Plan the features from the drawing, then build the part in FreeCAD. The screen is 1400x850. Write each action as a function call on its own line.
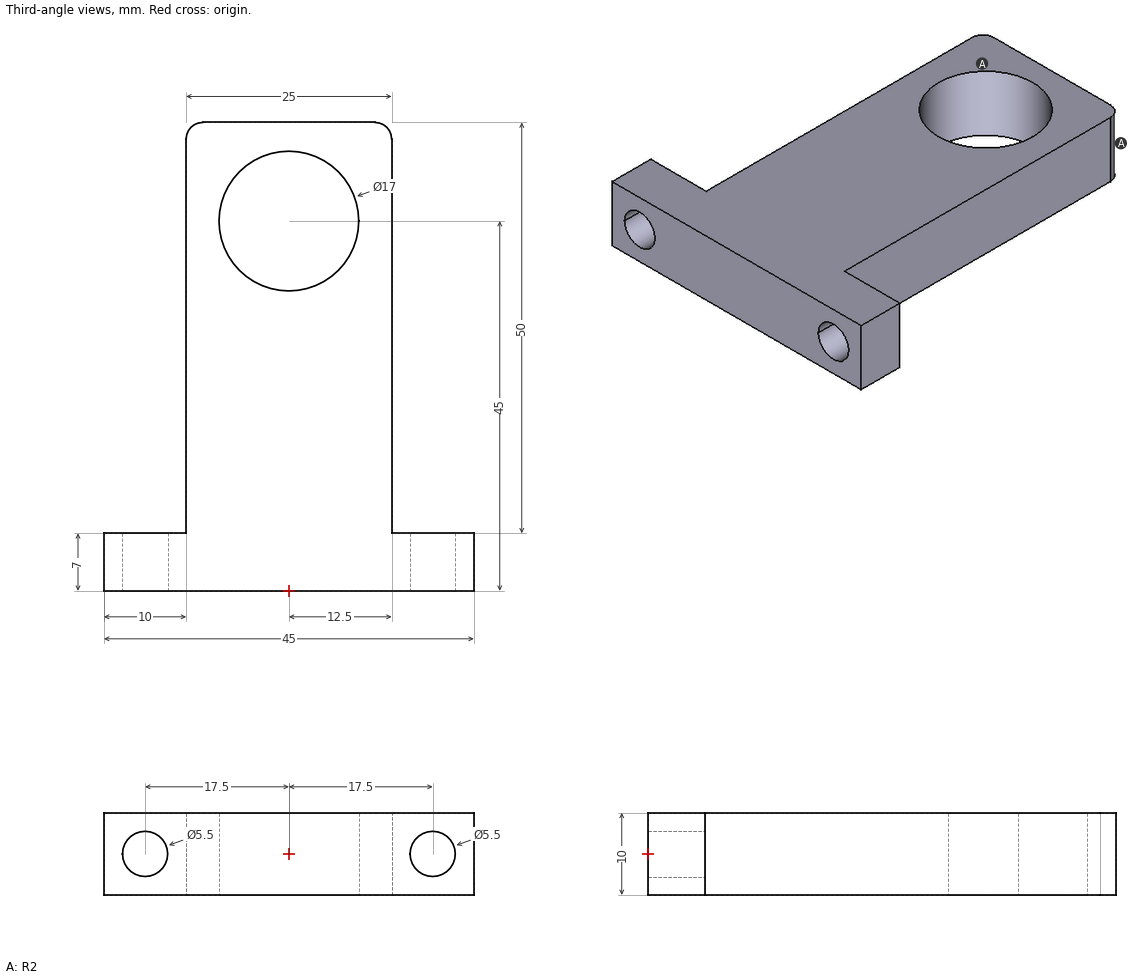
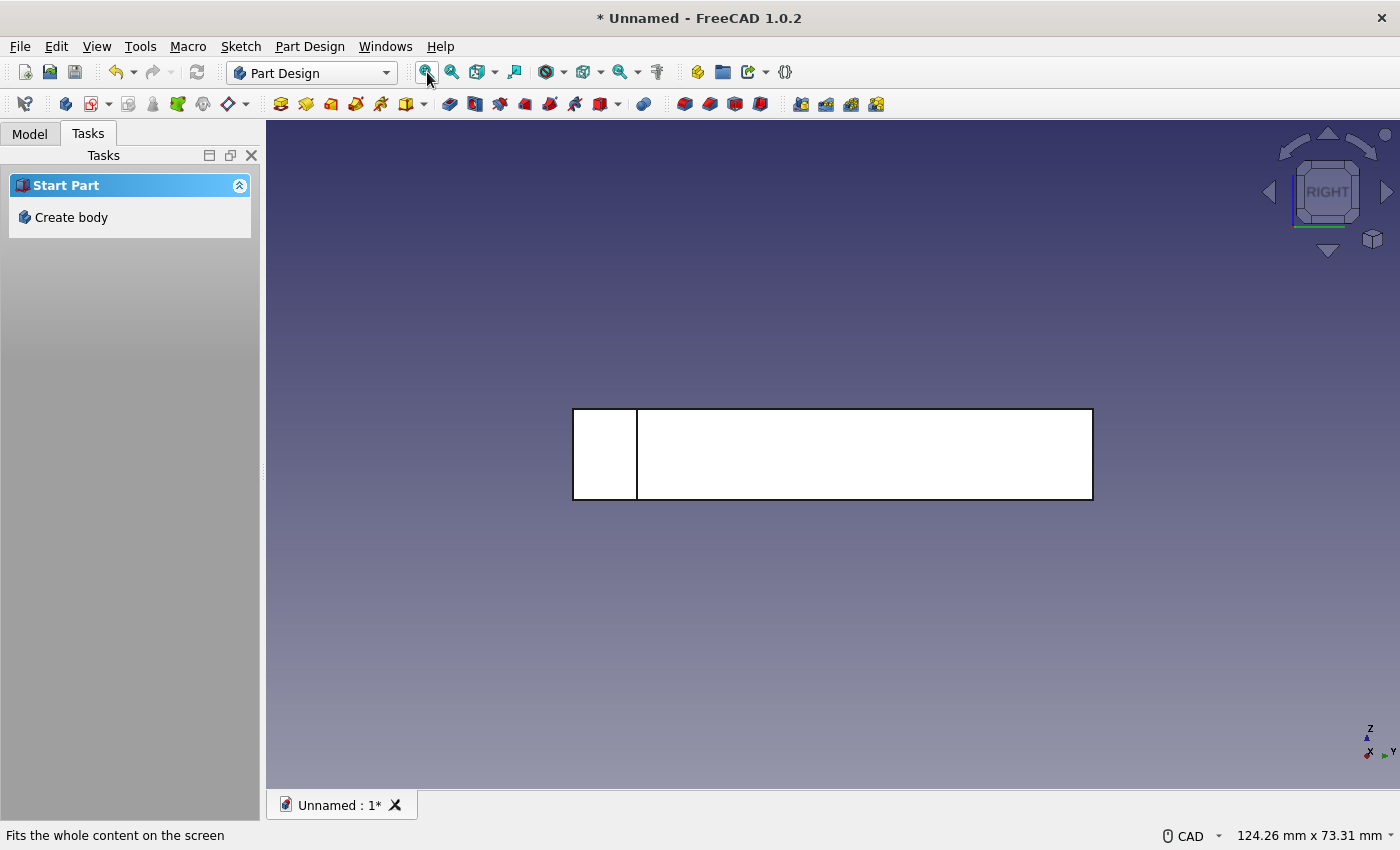
click(1093, 453)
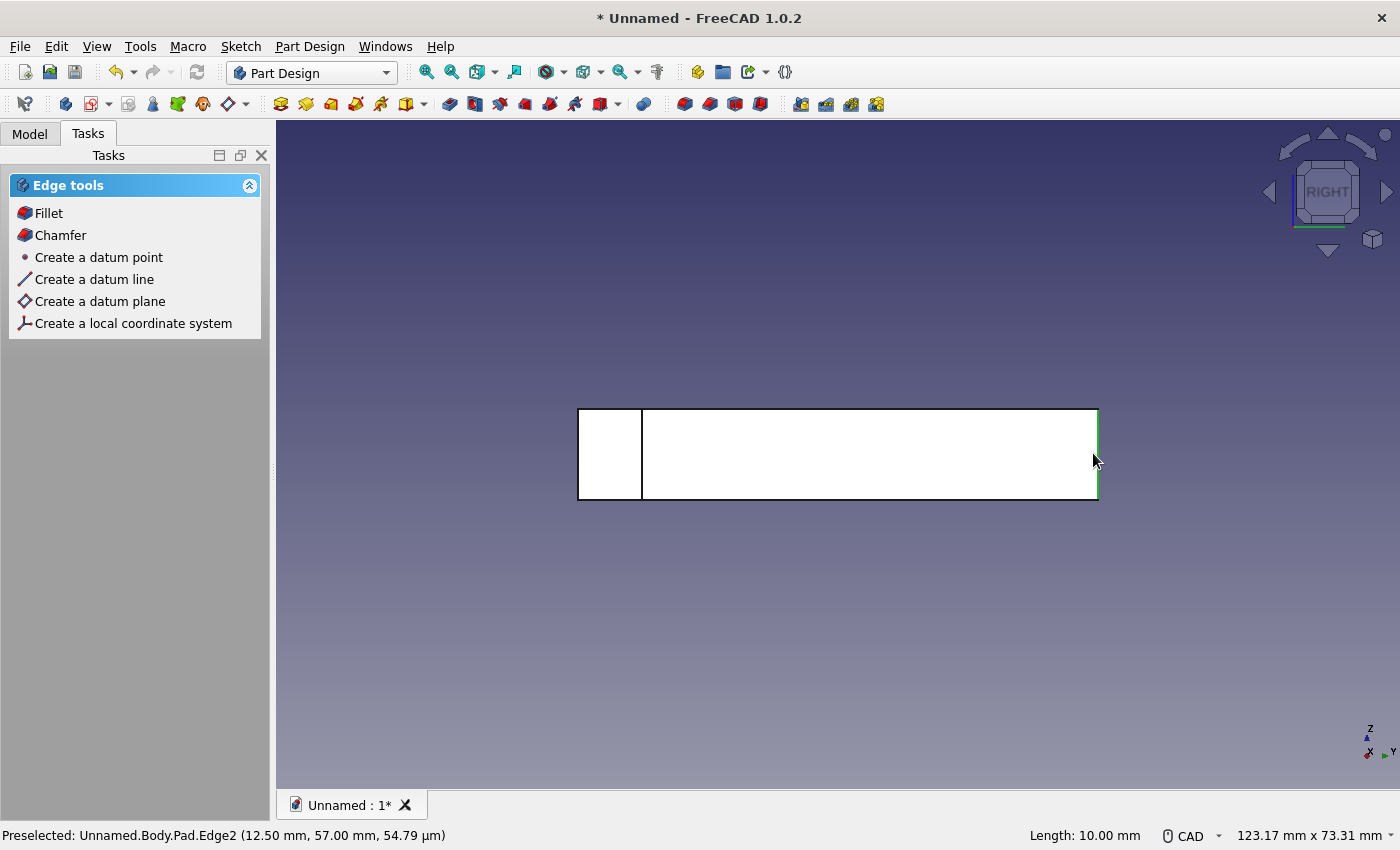
key(5)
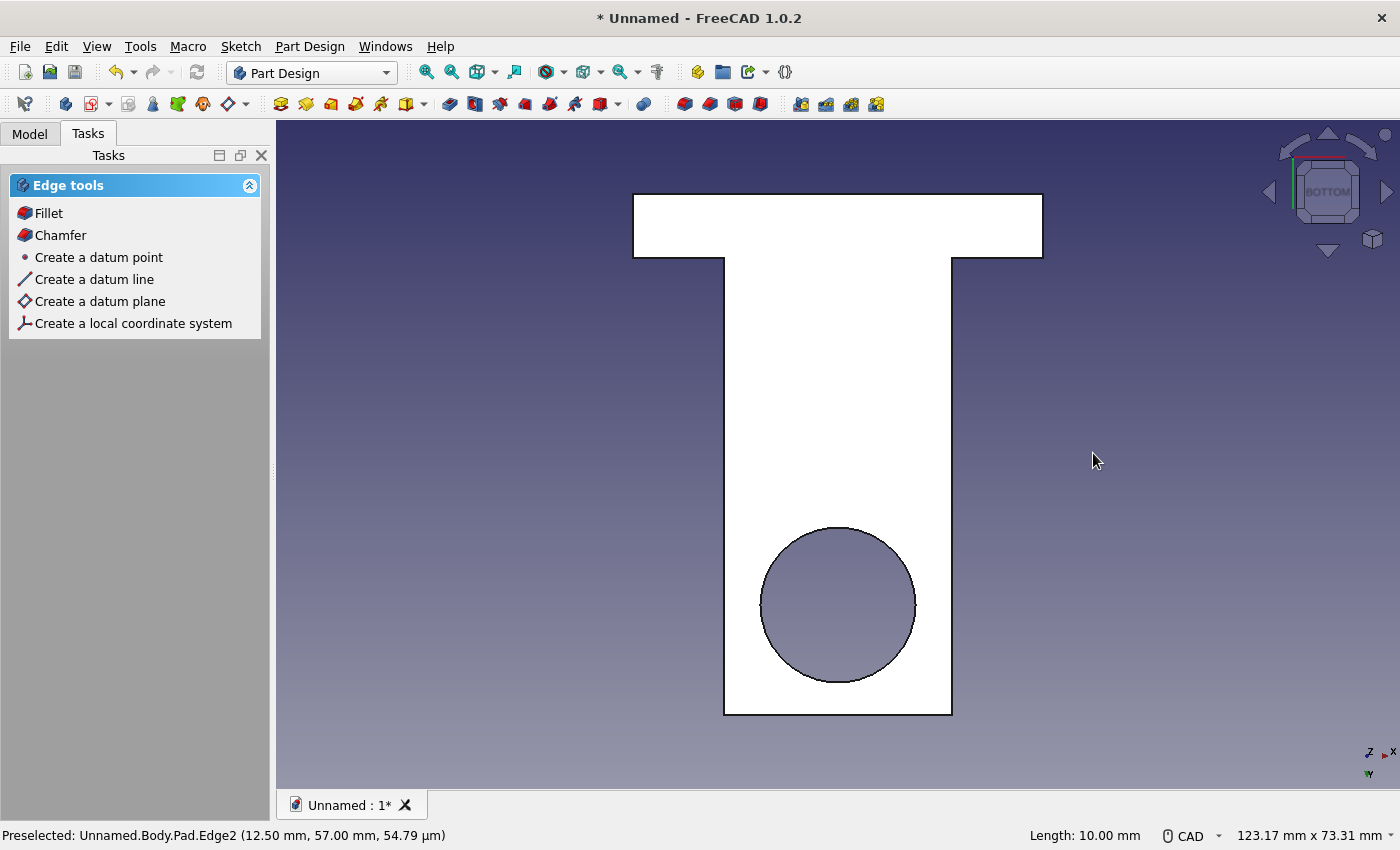
key(4)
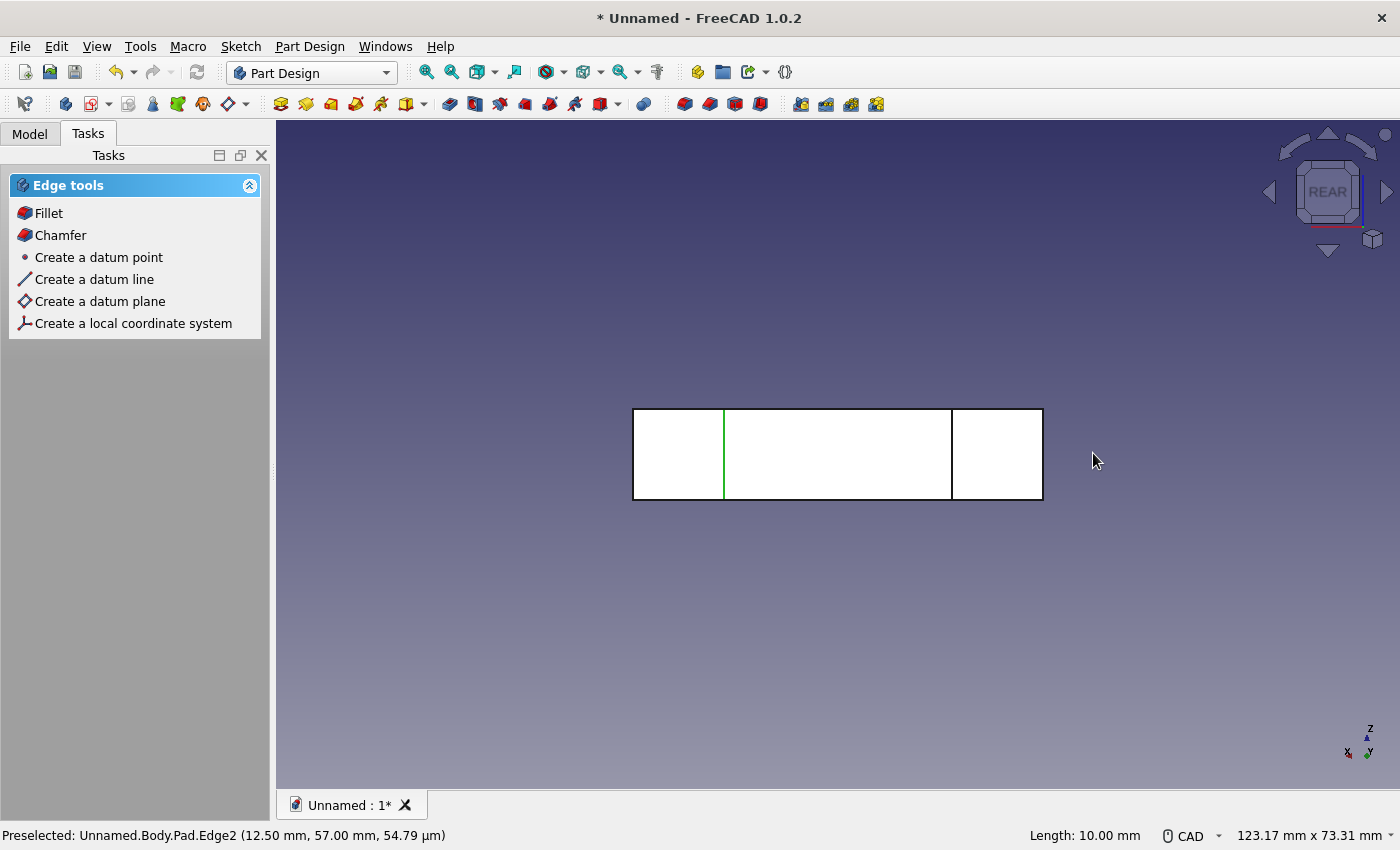
click(427, 72)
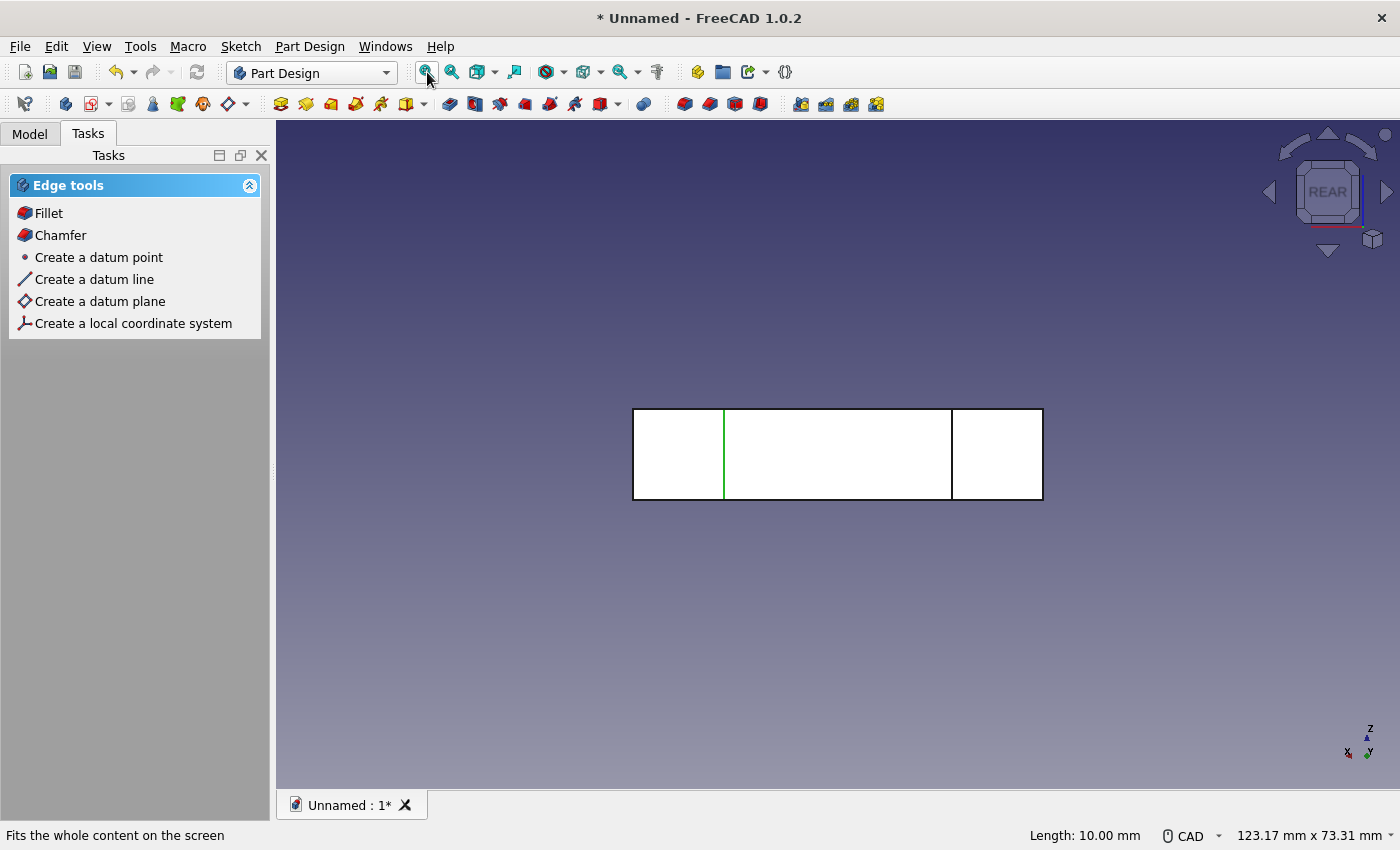
click(952, 454, ctrl)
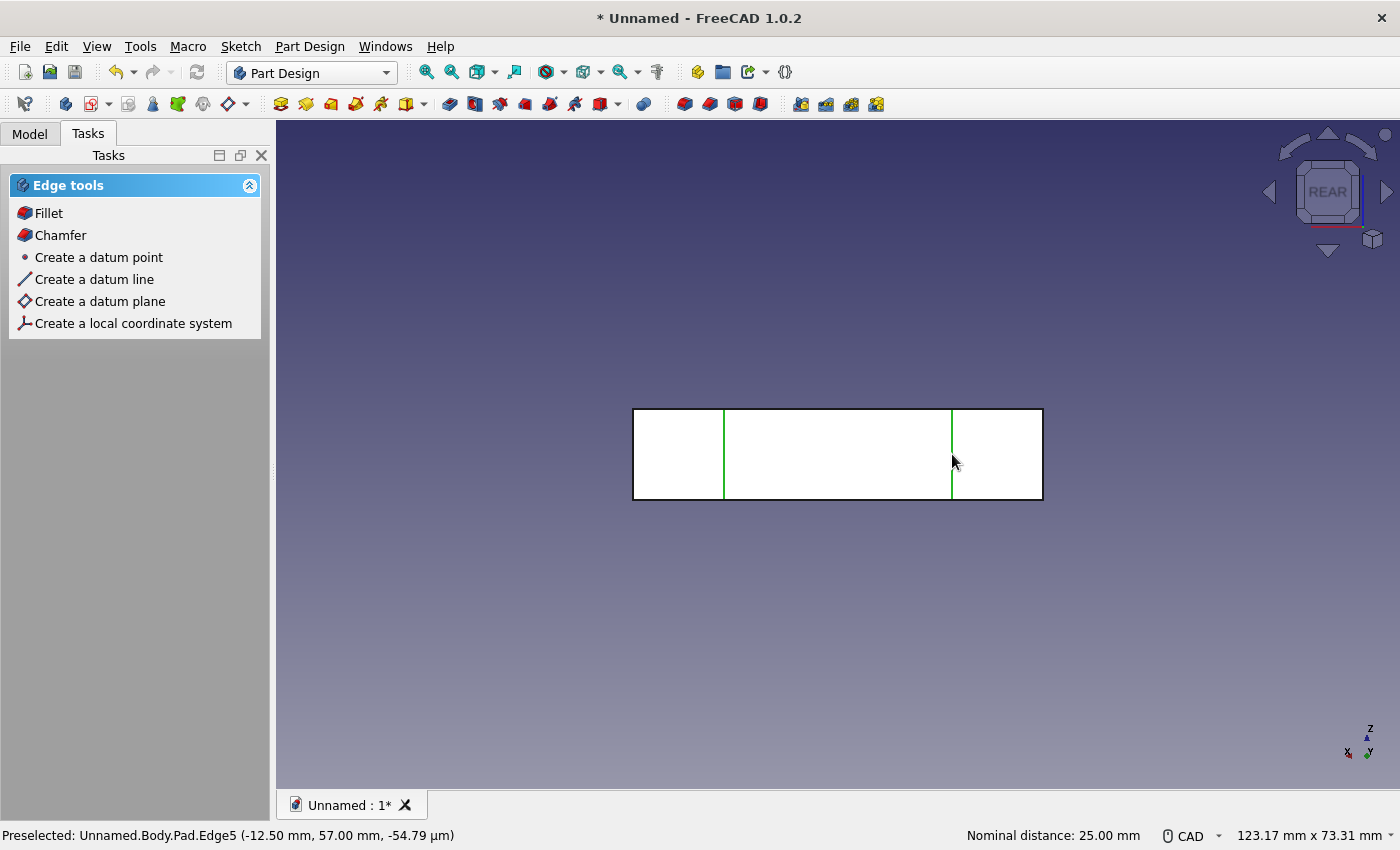
click(685, 104)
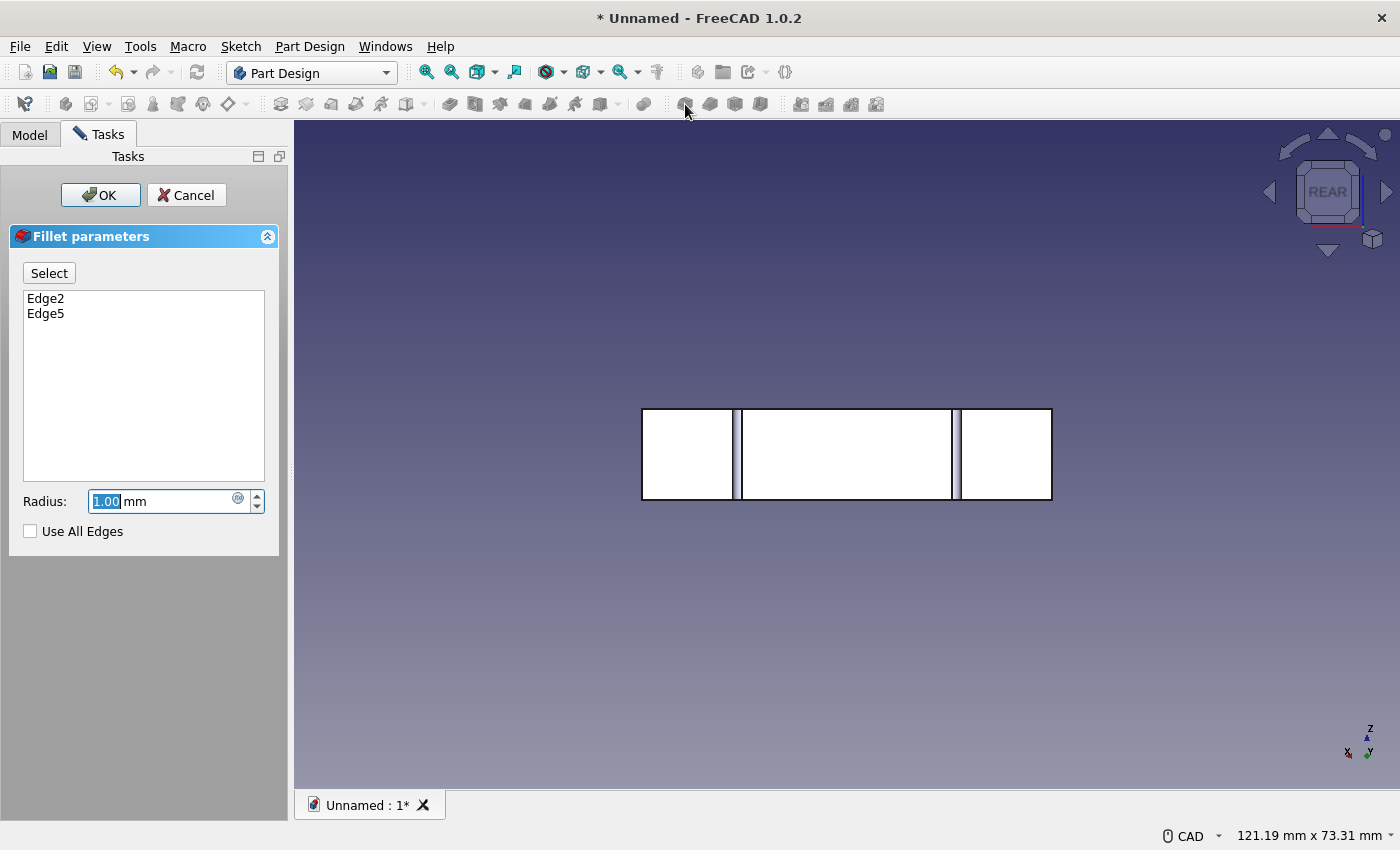
text(2)
key(Tab)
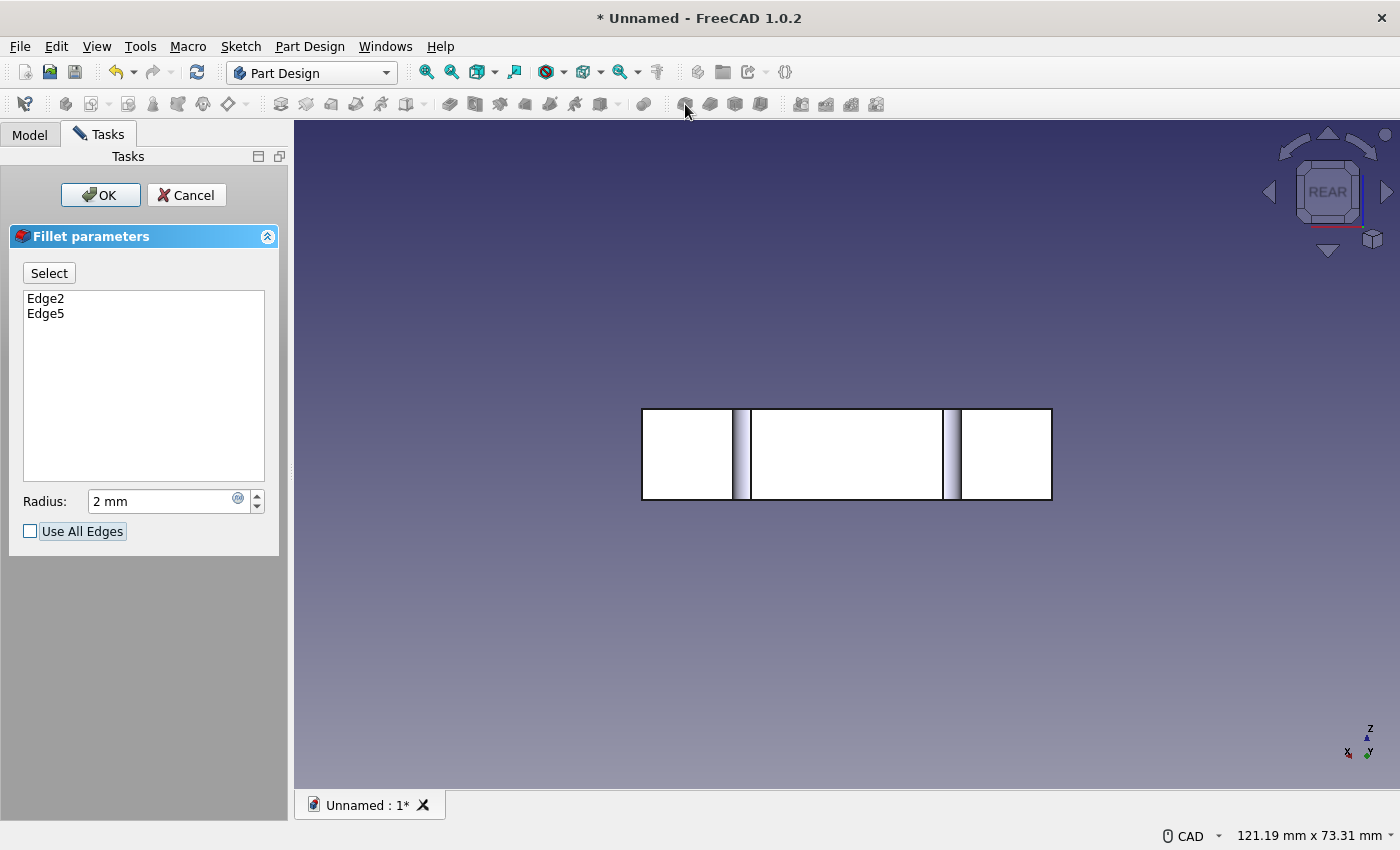
click(101, 195)